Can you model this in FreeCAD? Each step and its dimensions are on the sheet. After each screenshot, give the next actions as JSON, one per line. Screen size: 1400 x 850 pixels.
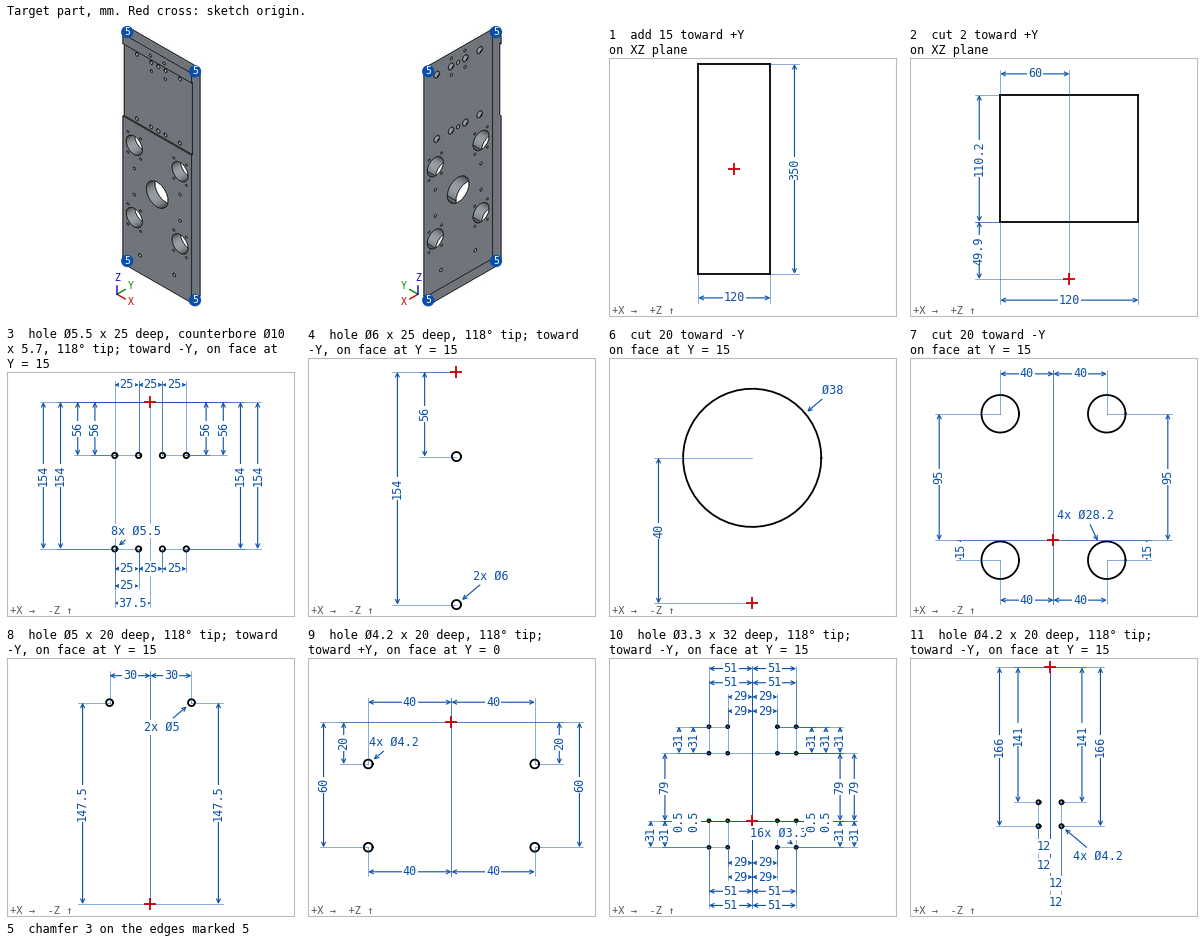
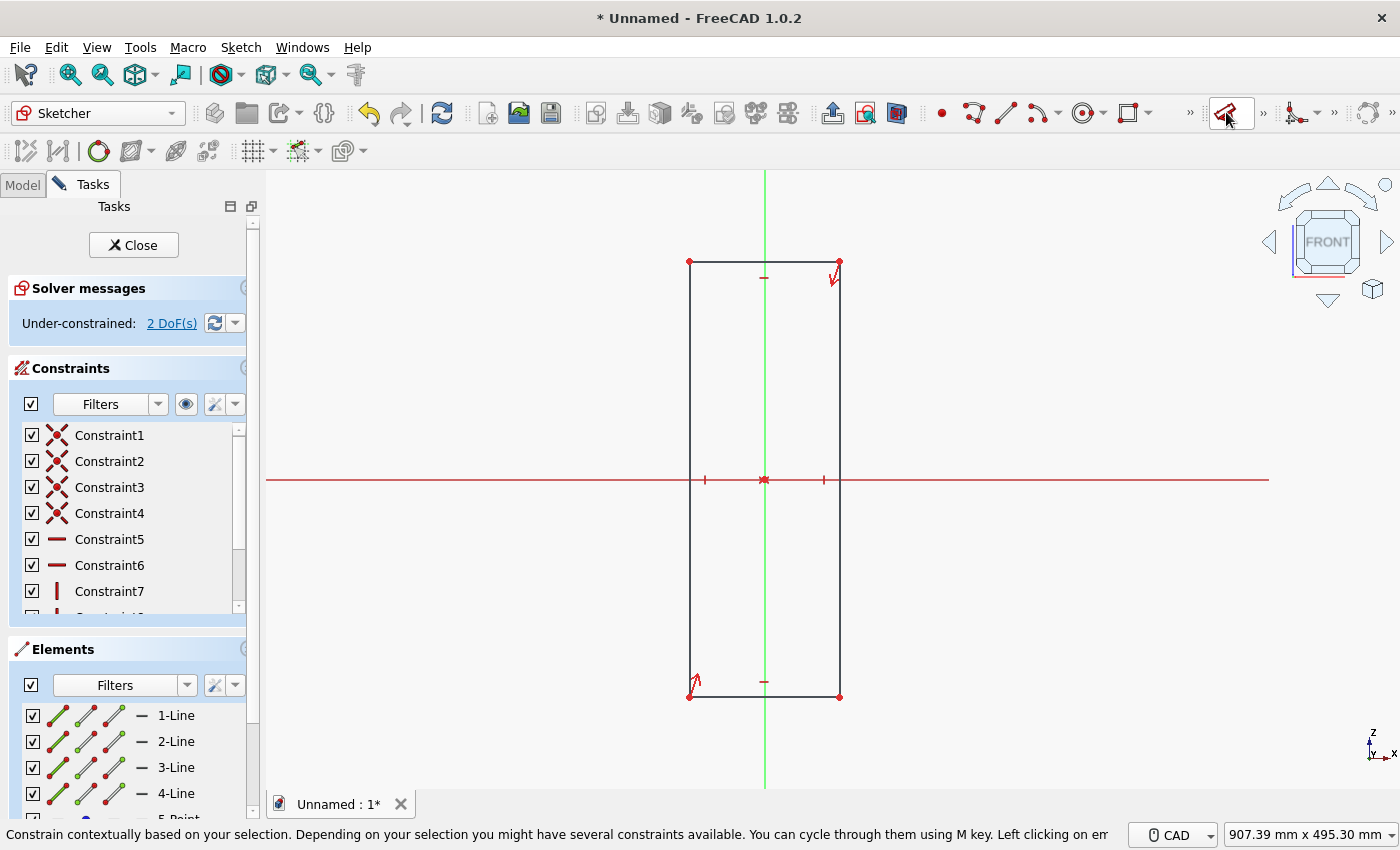
{"action": "left_click", "coordinate": [735, 697]}
{"action": "left_click", "coordinate": [730, 731]}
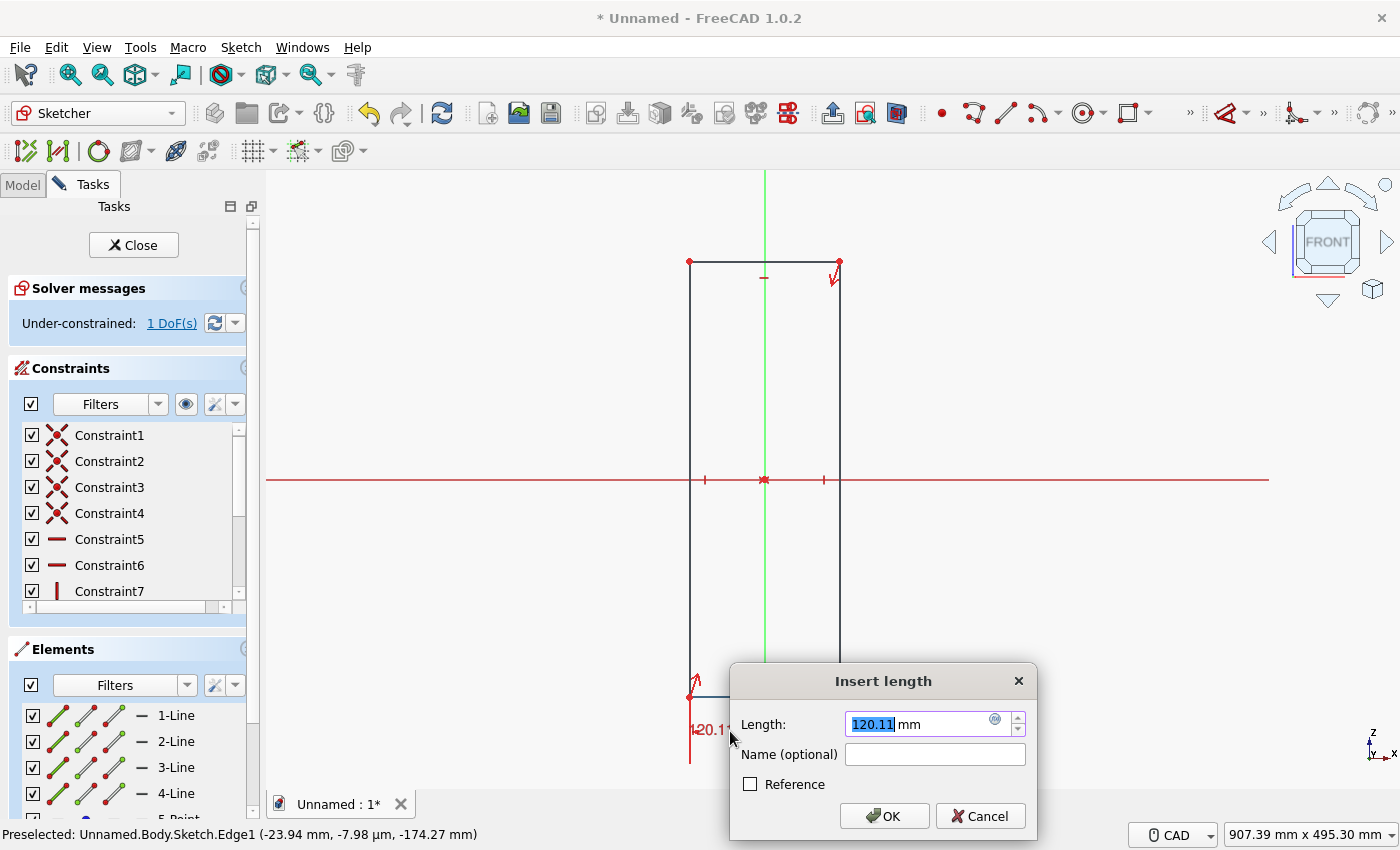
{"action": "type", "text": "120"}
{"action": "key", "text": "Return"}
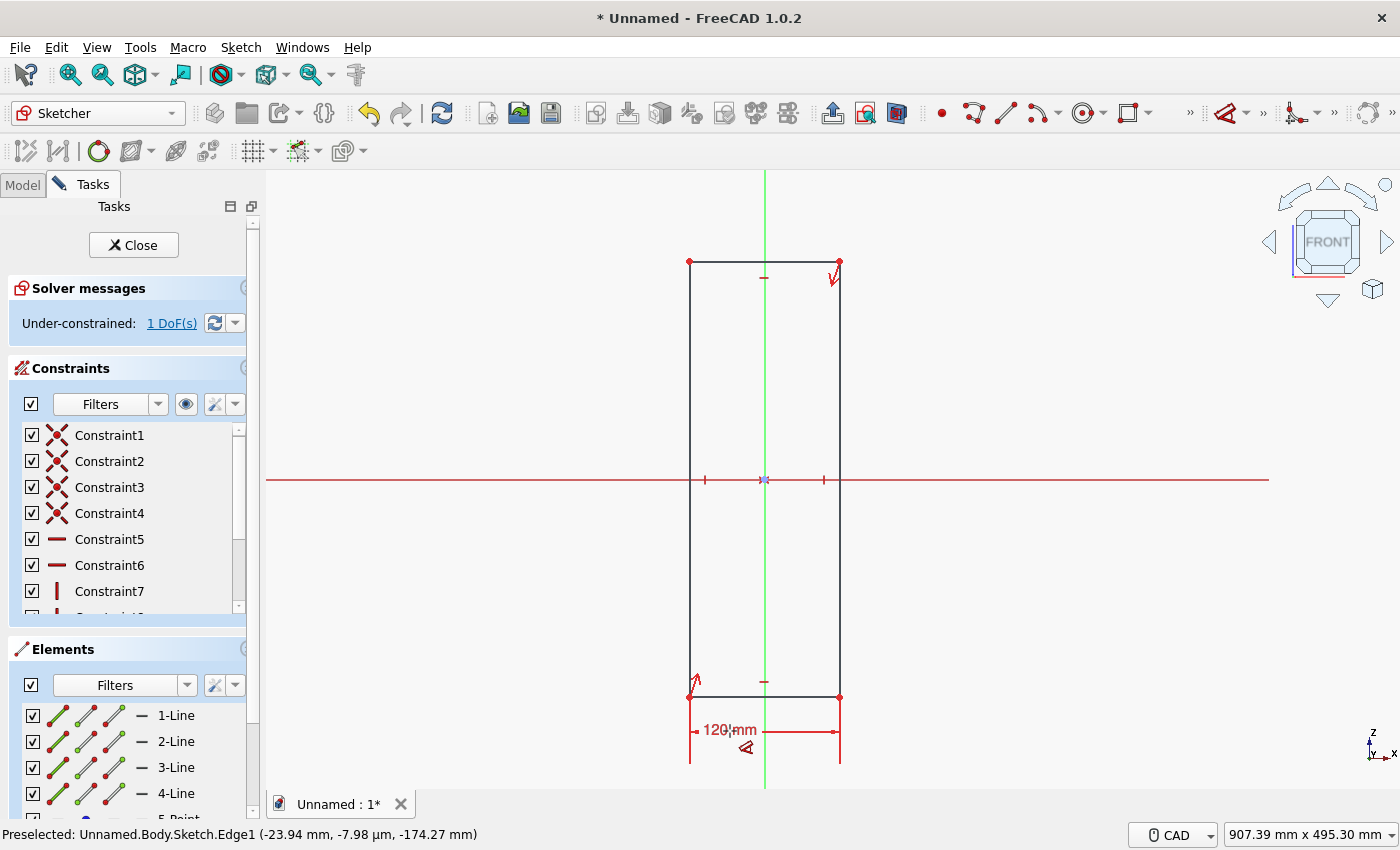
{"action": "left_click", "coordinate": [840, 567]}
{"action": "left_click", "coordinate": [874, 379]}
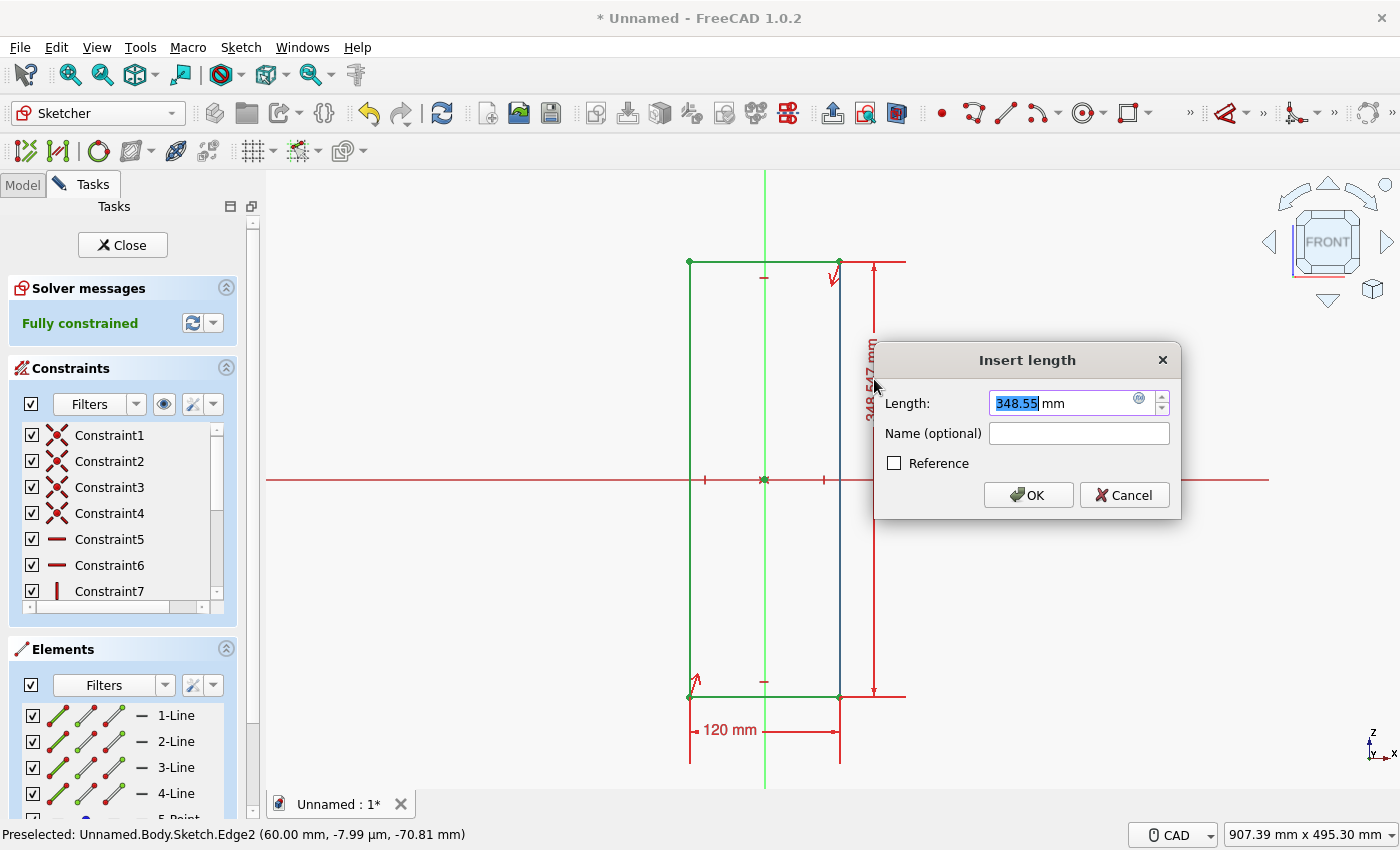
{"action": "type", "text": "350"}
{"action": "key", "text": "Return"}
{"action": "key", "text": "Escape"}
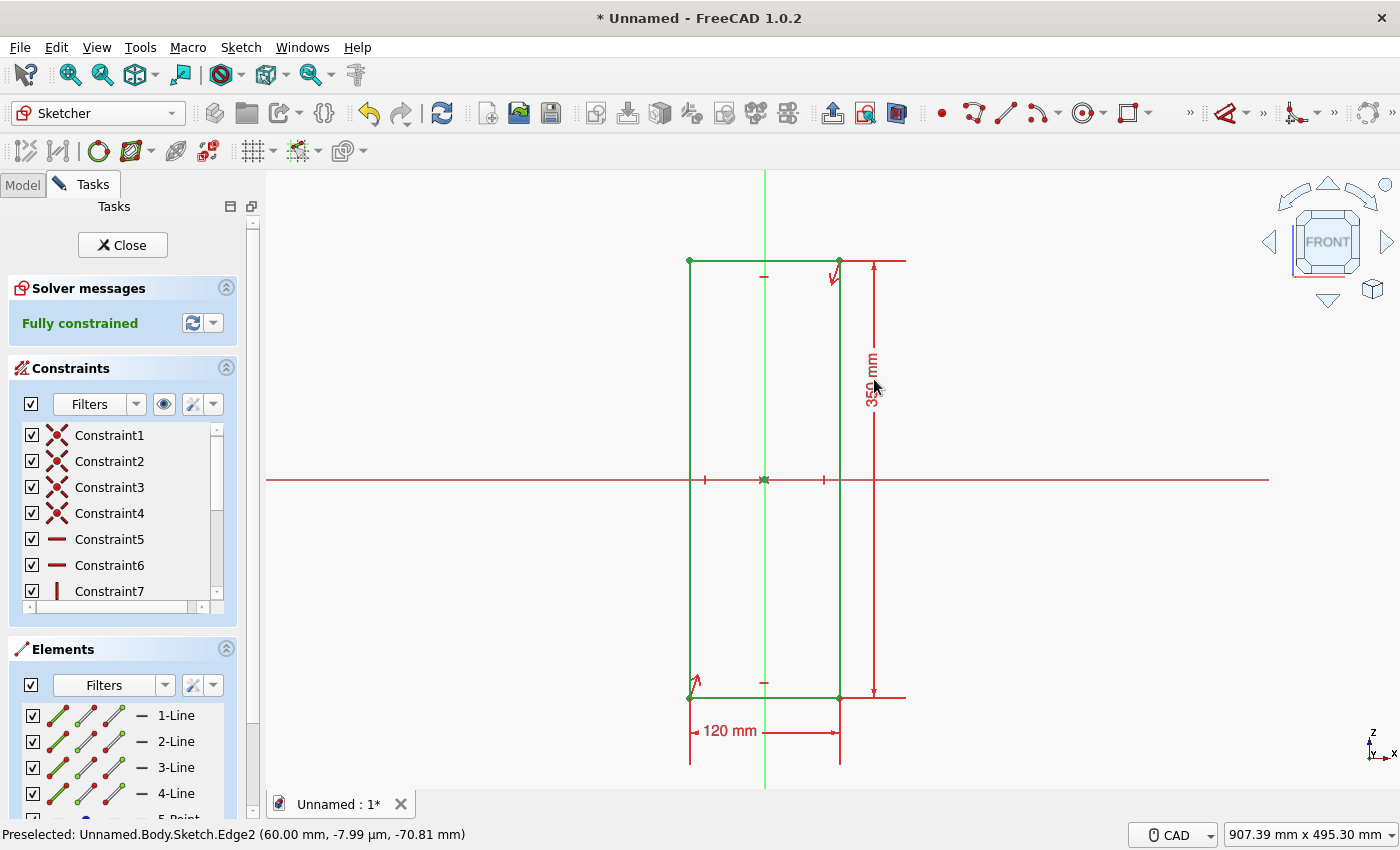
{"action": "left_click", "coordinate": [123, 245]}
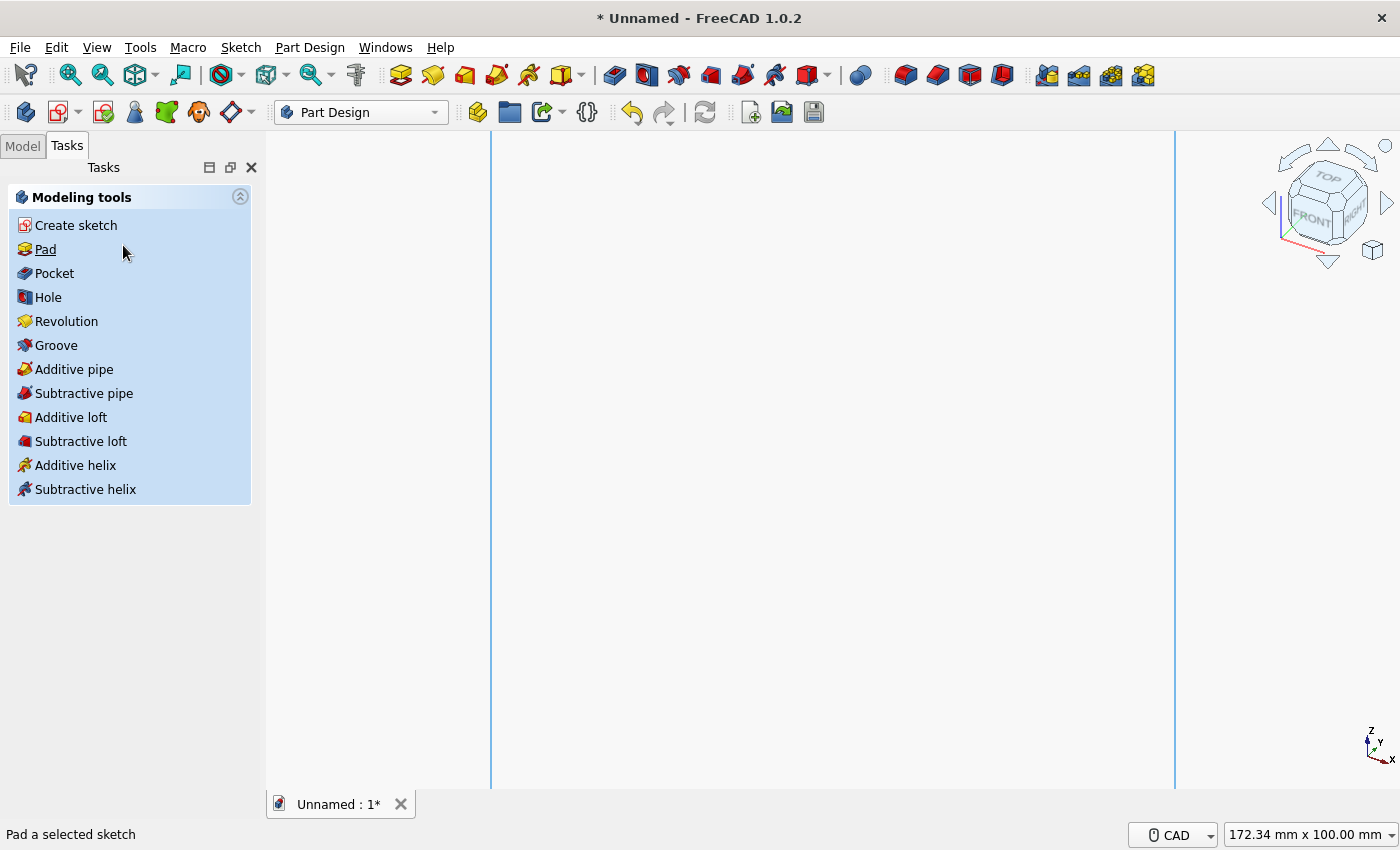
{"action": "left_click", "coordinate": [402, 76]}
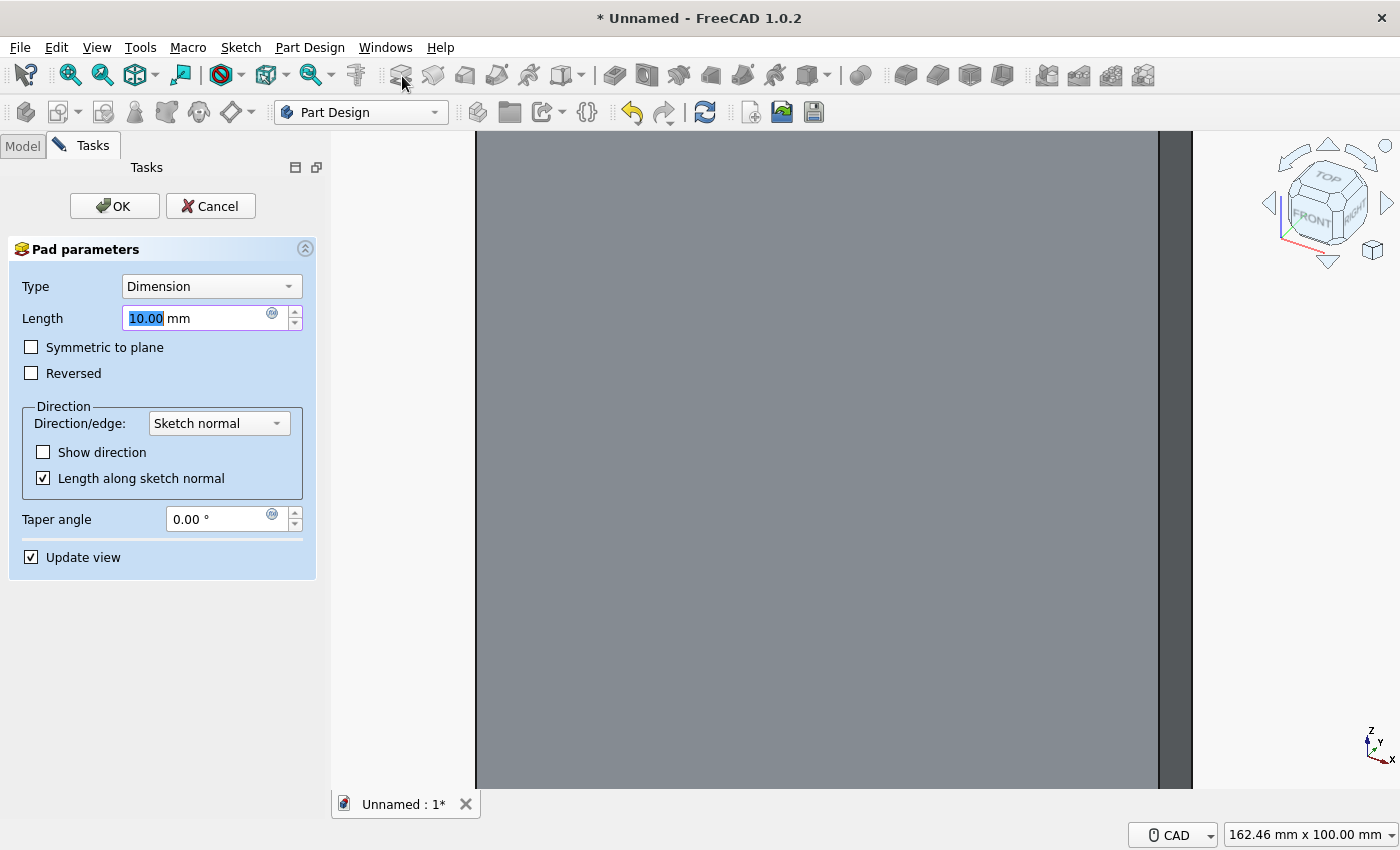
{"action": "type", "text": "15"}
{"action": "key", "text": "Tab"}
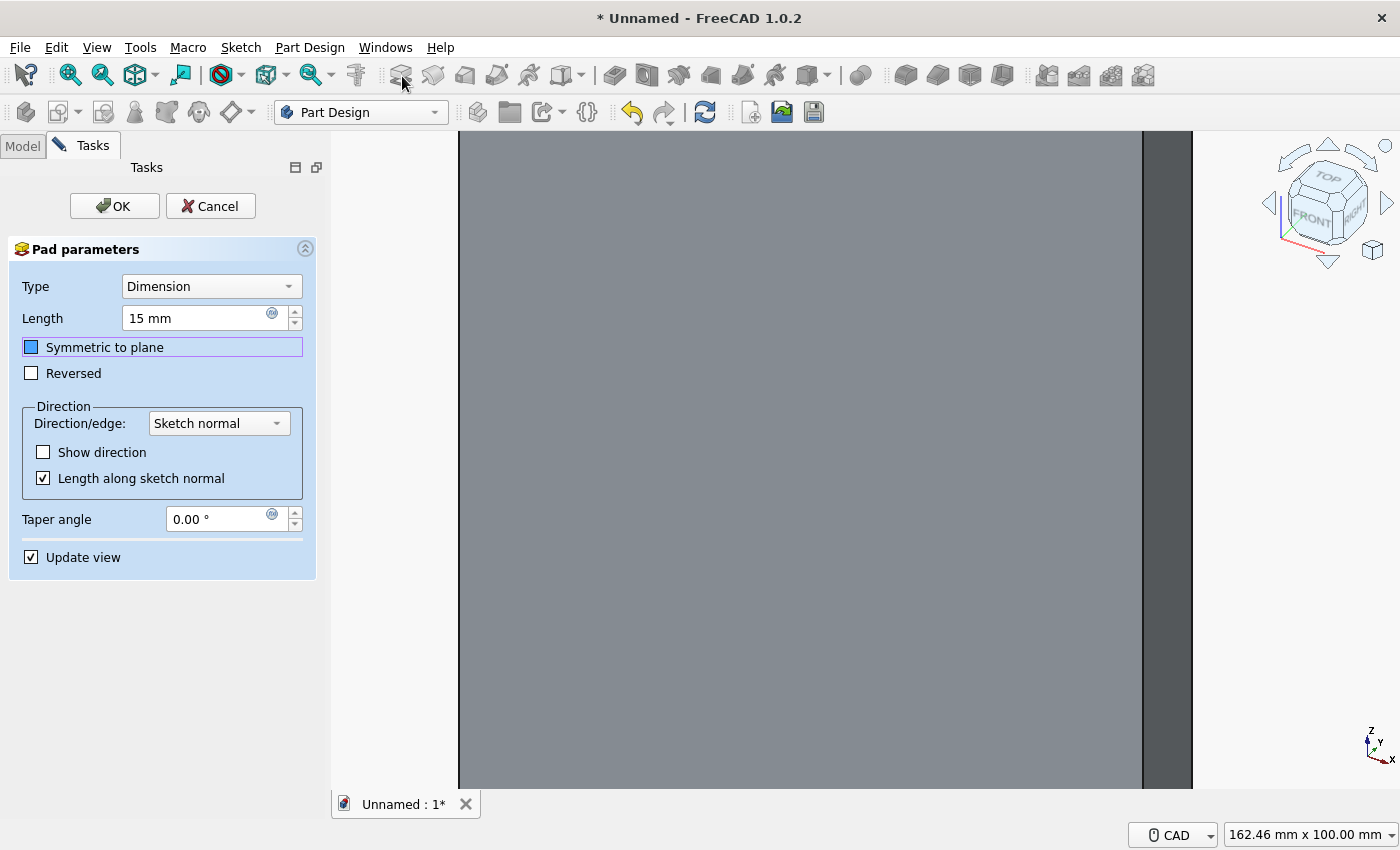
{"action": "left_click", "coordinate": [30, 373]}